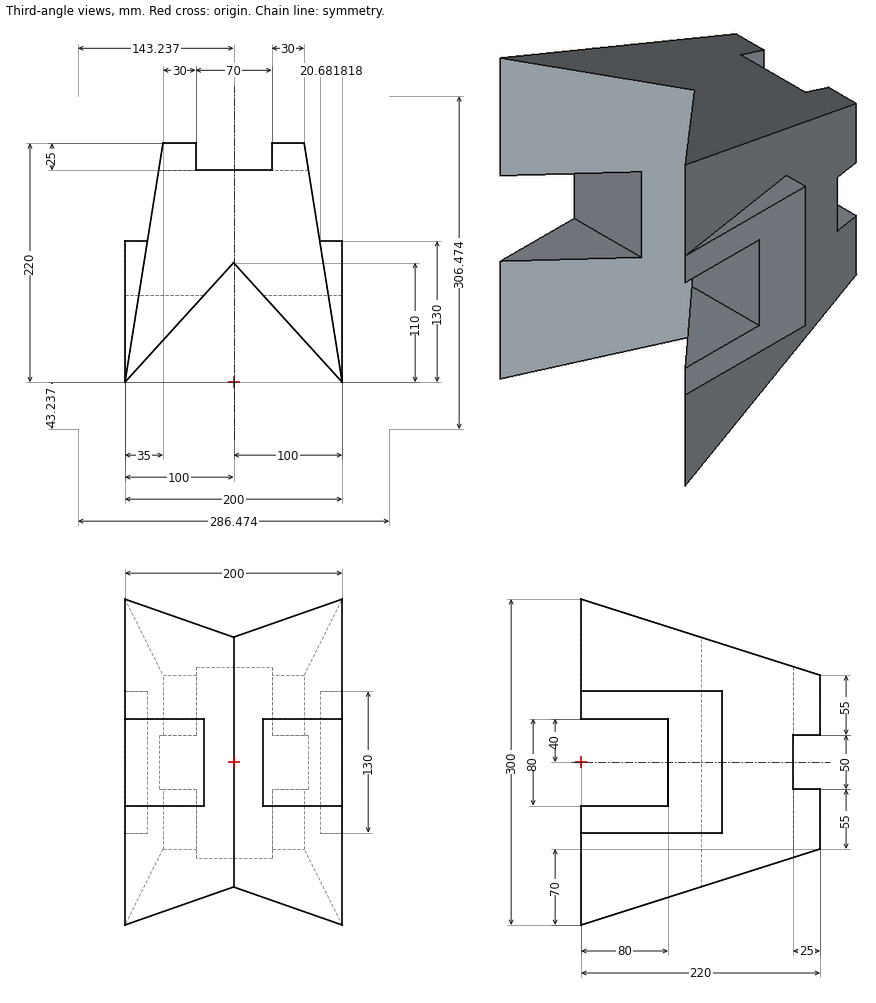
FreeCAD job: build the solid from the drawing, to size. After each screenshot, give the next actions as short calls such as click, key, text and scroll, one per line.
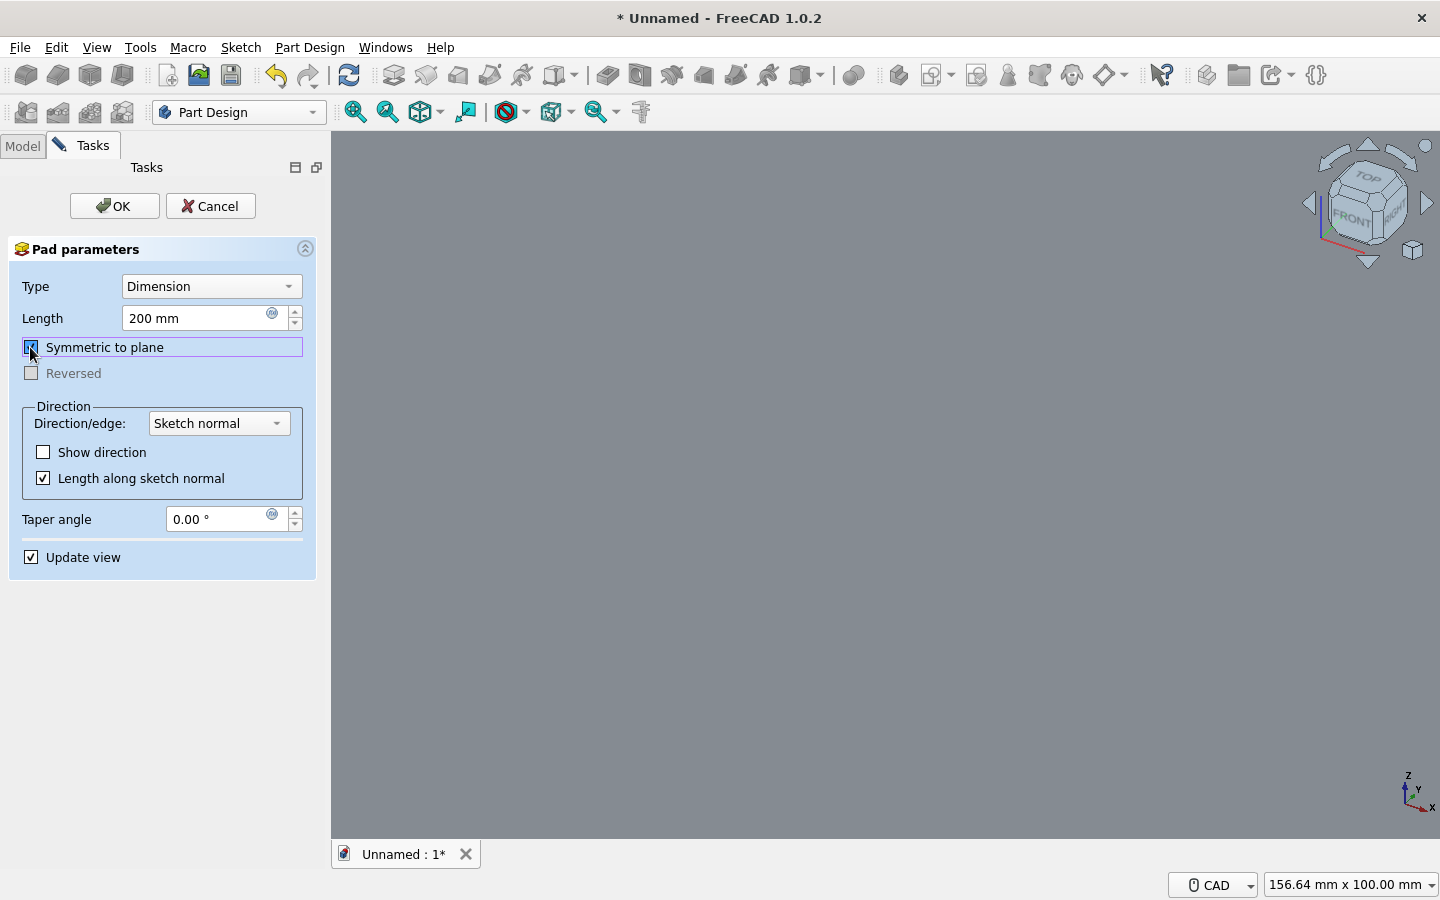
click(115, 206)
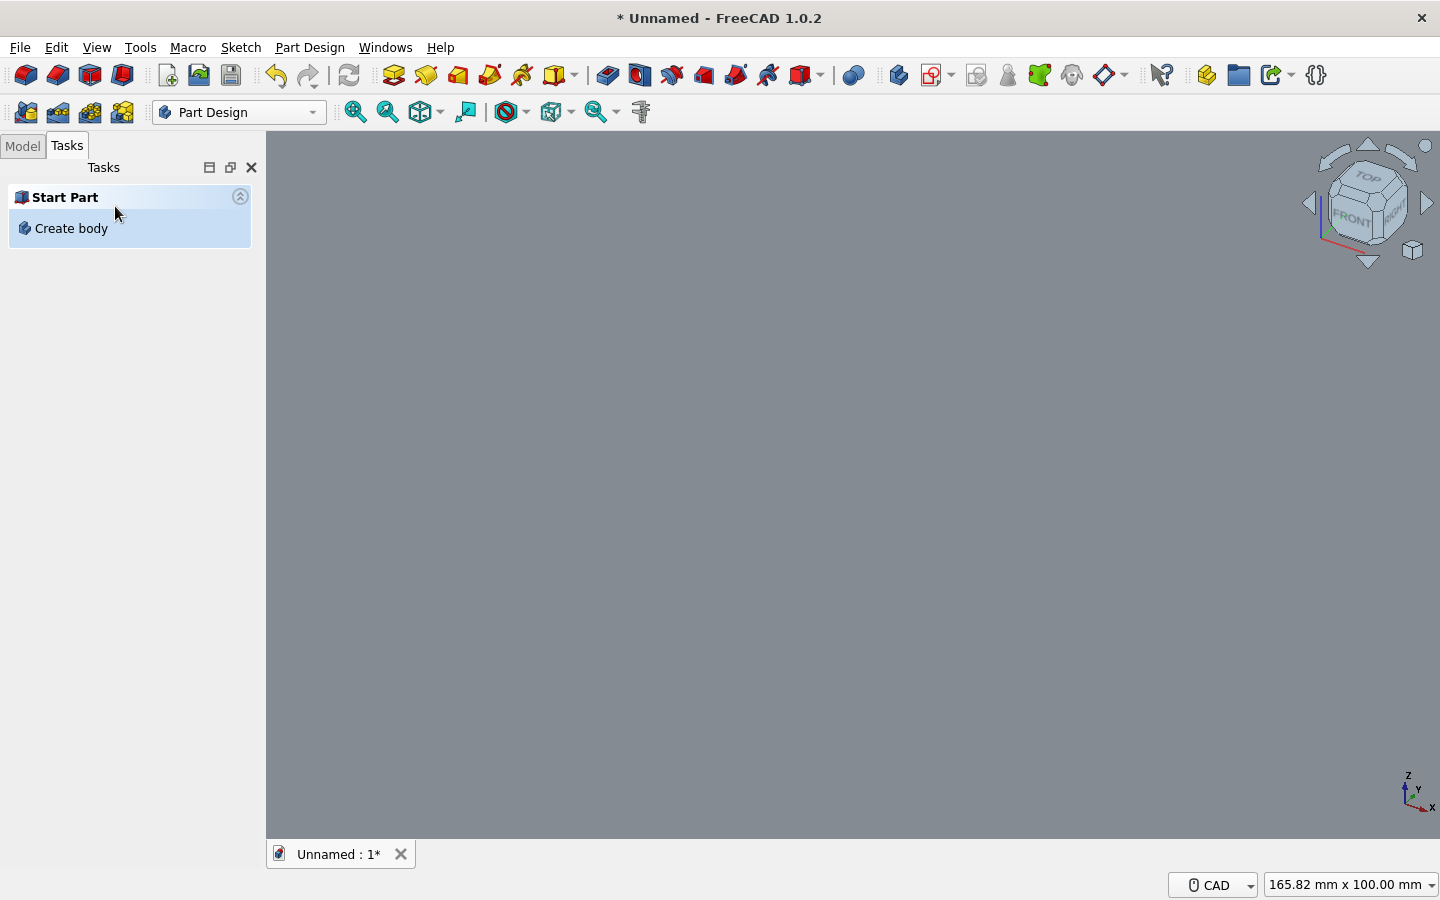
key(v)
key(f)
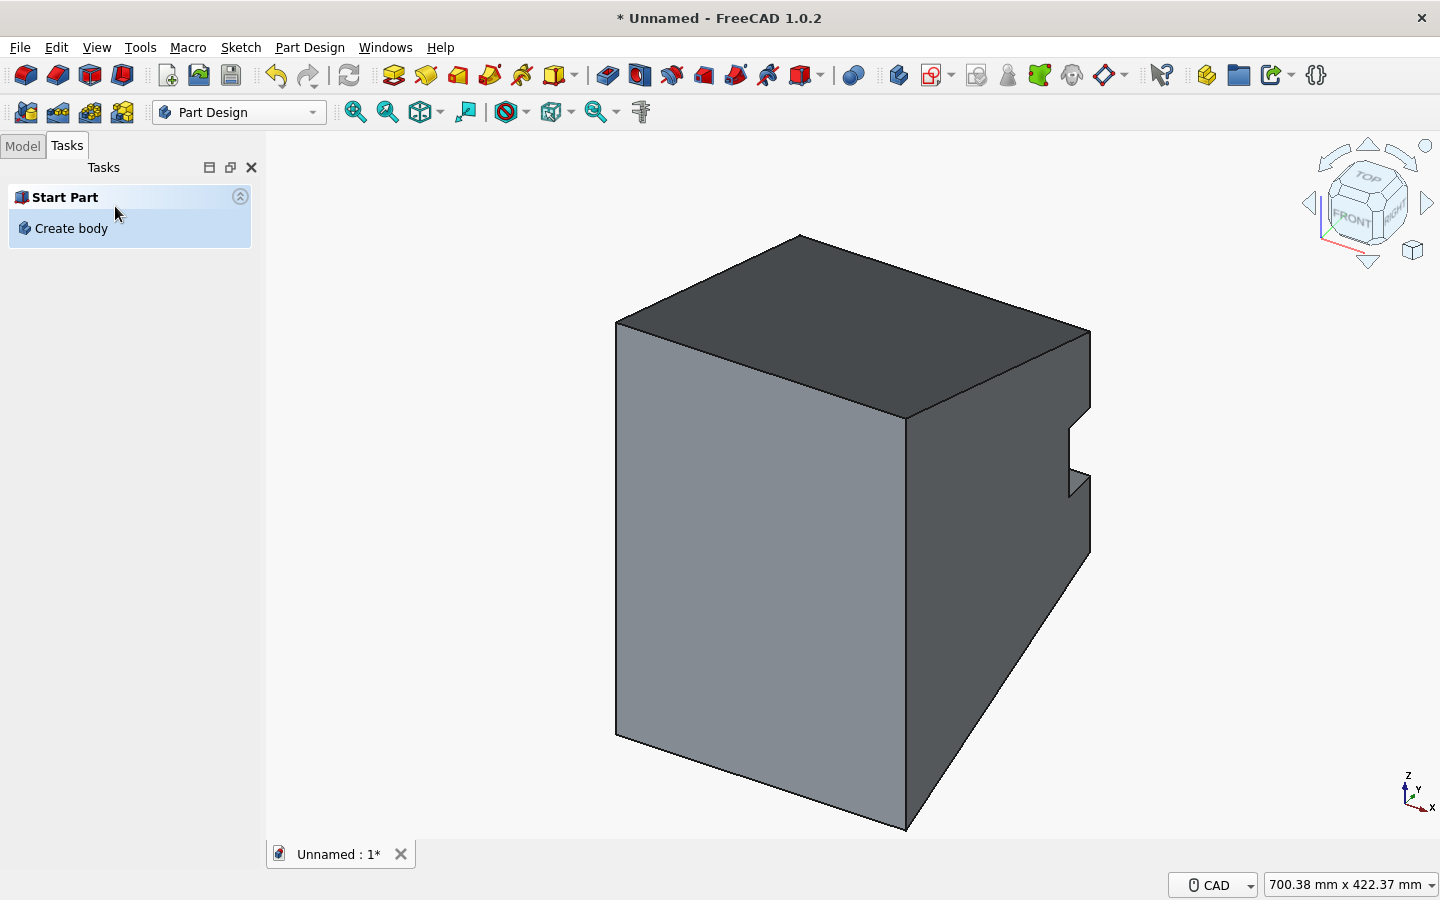
click(932, 76)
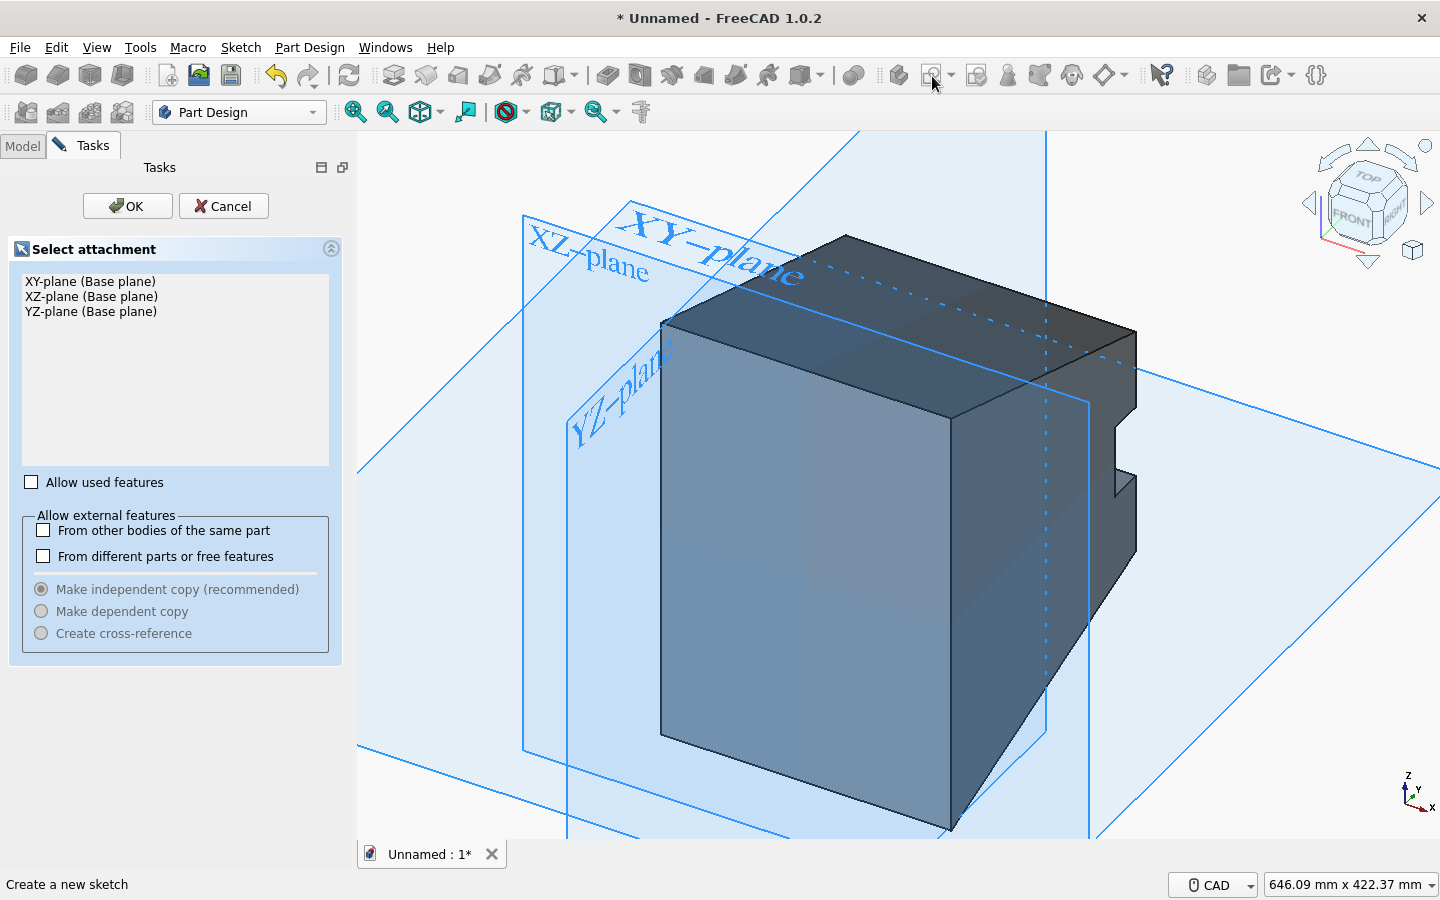
click(82, 282)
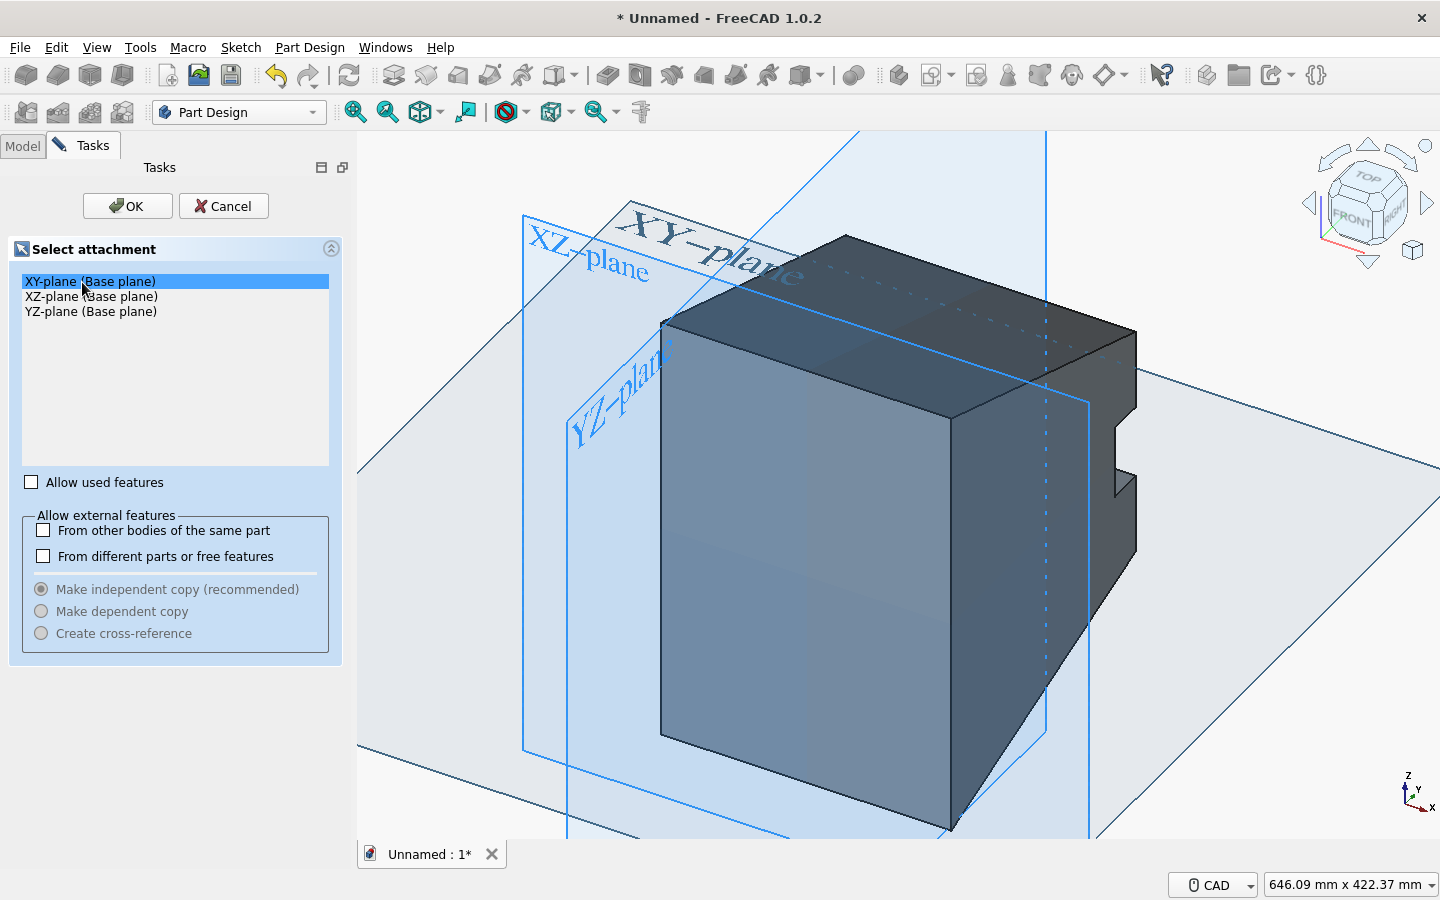
click(128, 206)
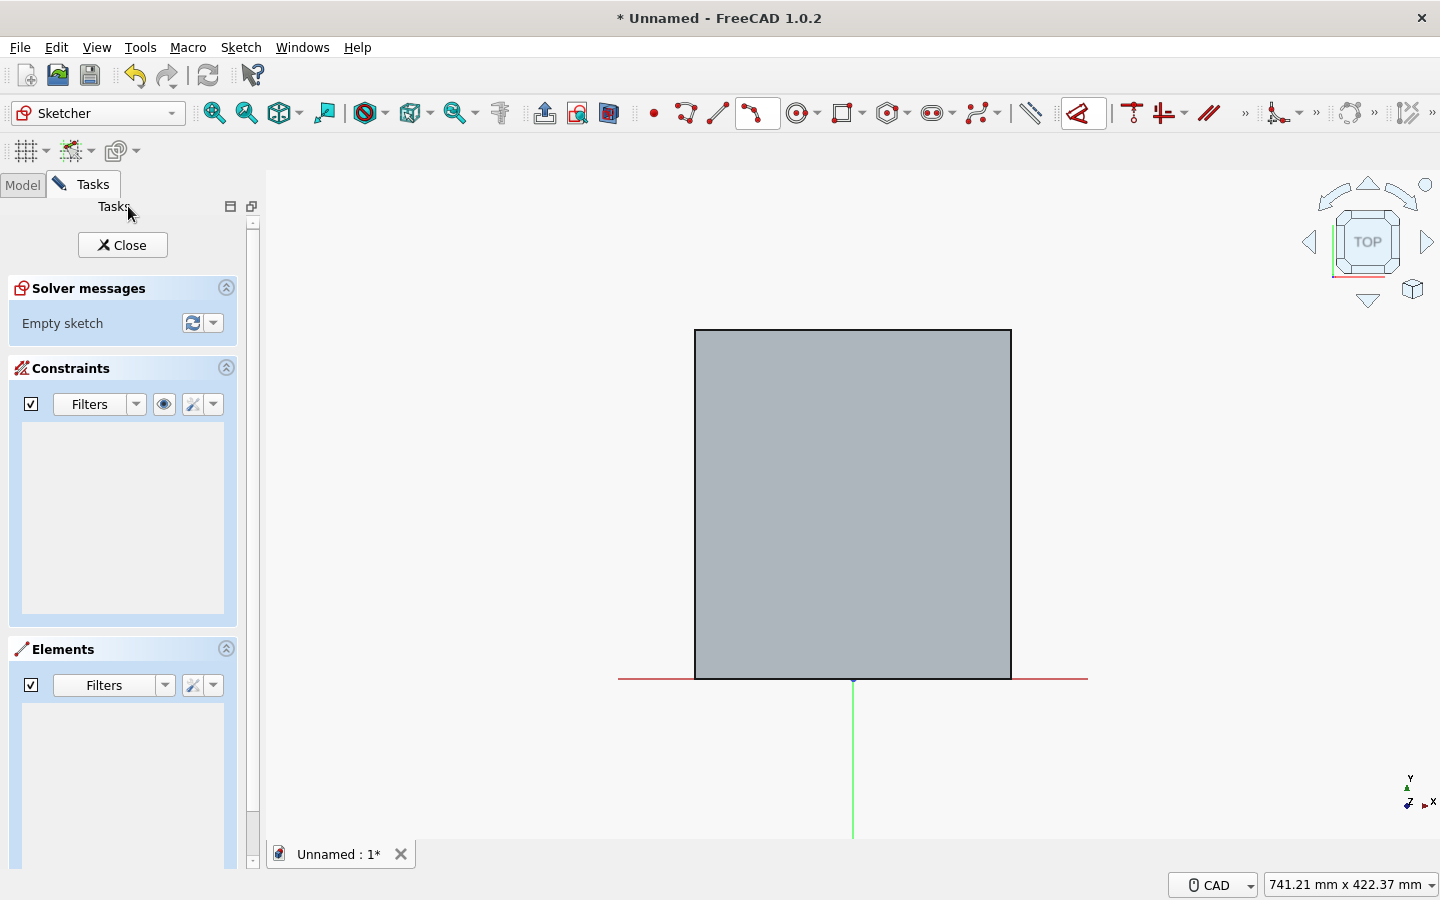
key(q)
key(s)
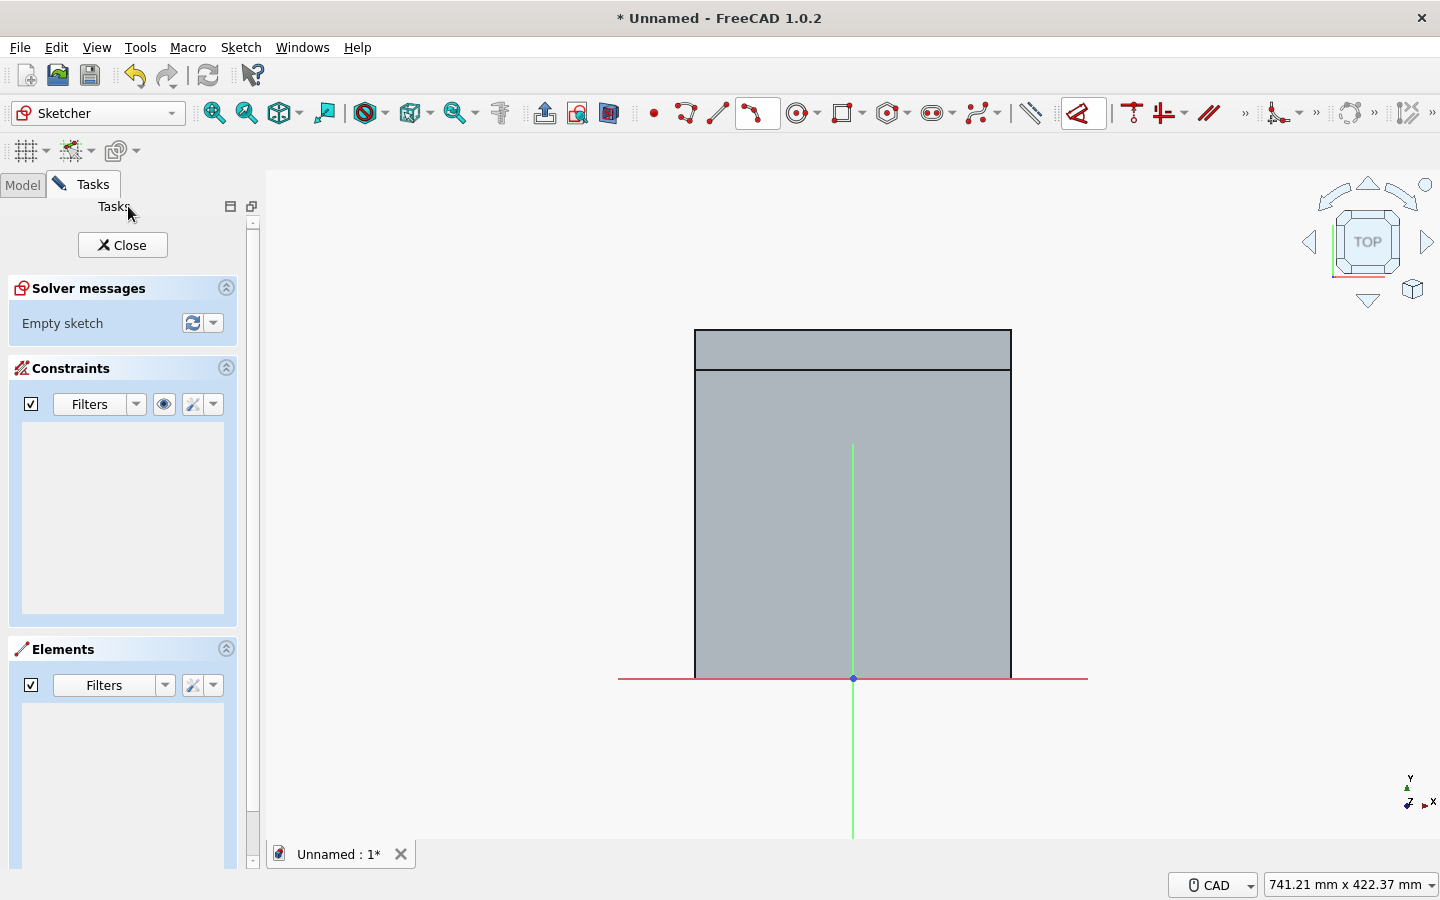
key(g)
key(r)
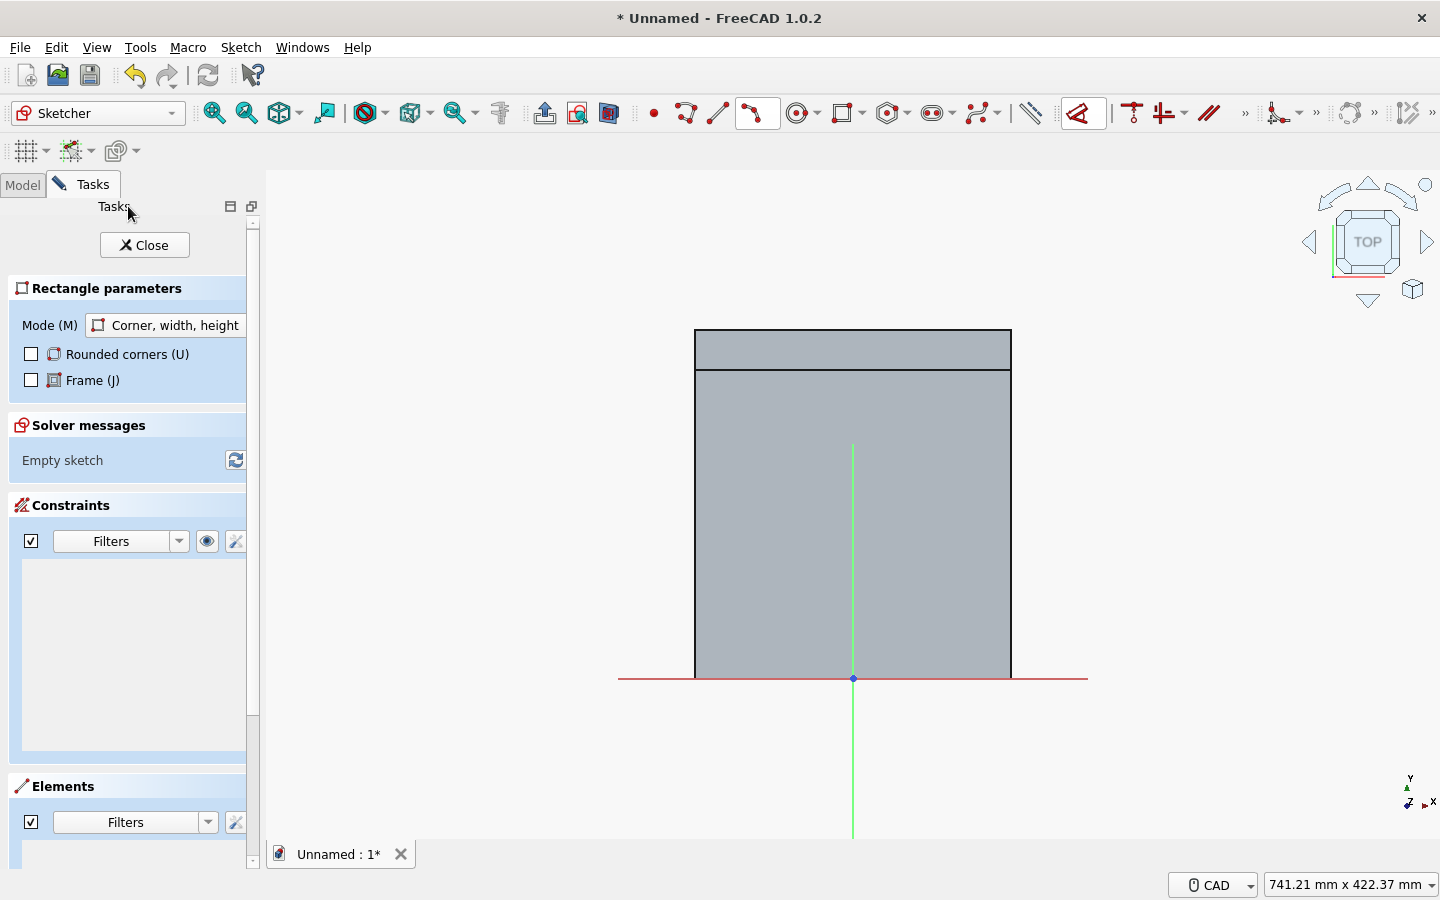
click(626, 262)
move(1080, 747)